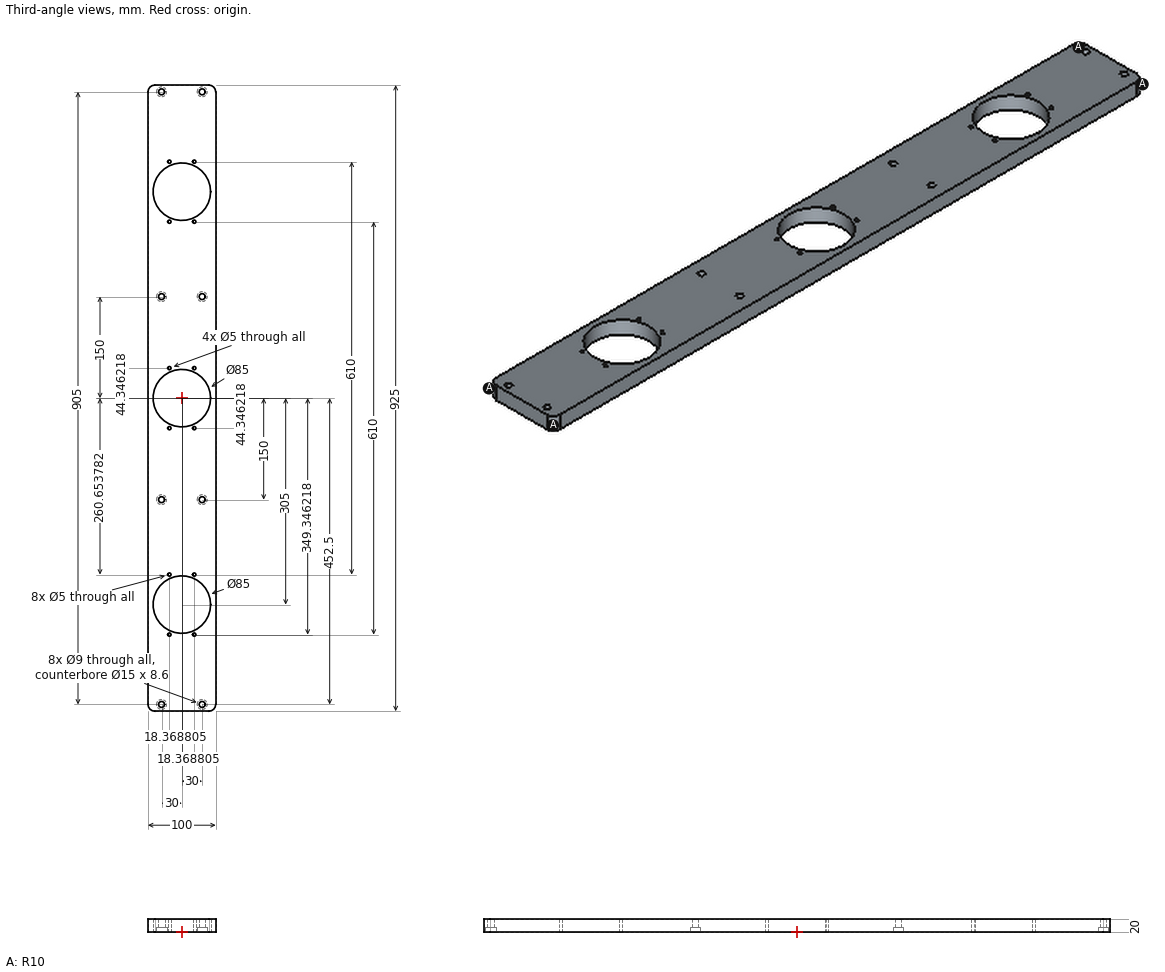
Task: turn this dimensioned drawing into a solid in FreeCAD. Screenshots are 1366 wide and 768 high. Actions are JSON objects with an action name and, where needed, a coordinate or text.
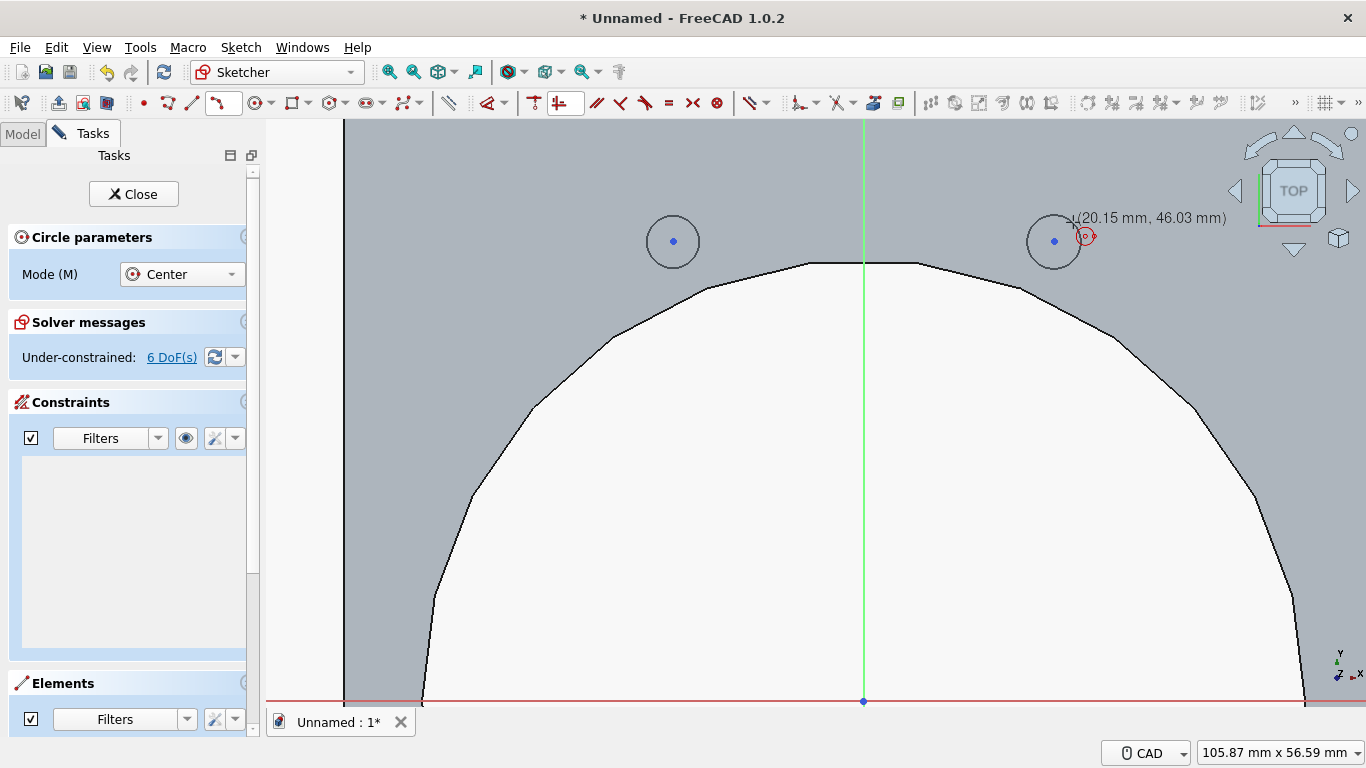
{"action": "scroll", "coordinate": [680, 245], "scroll_direction": "down", "scroll_amount": 5}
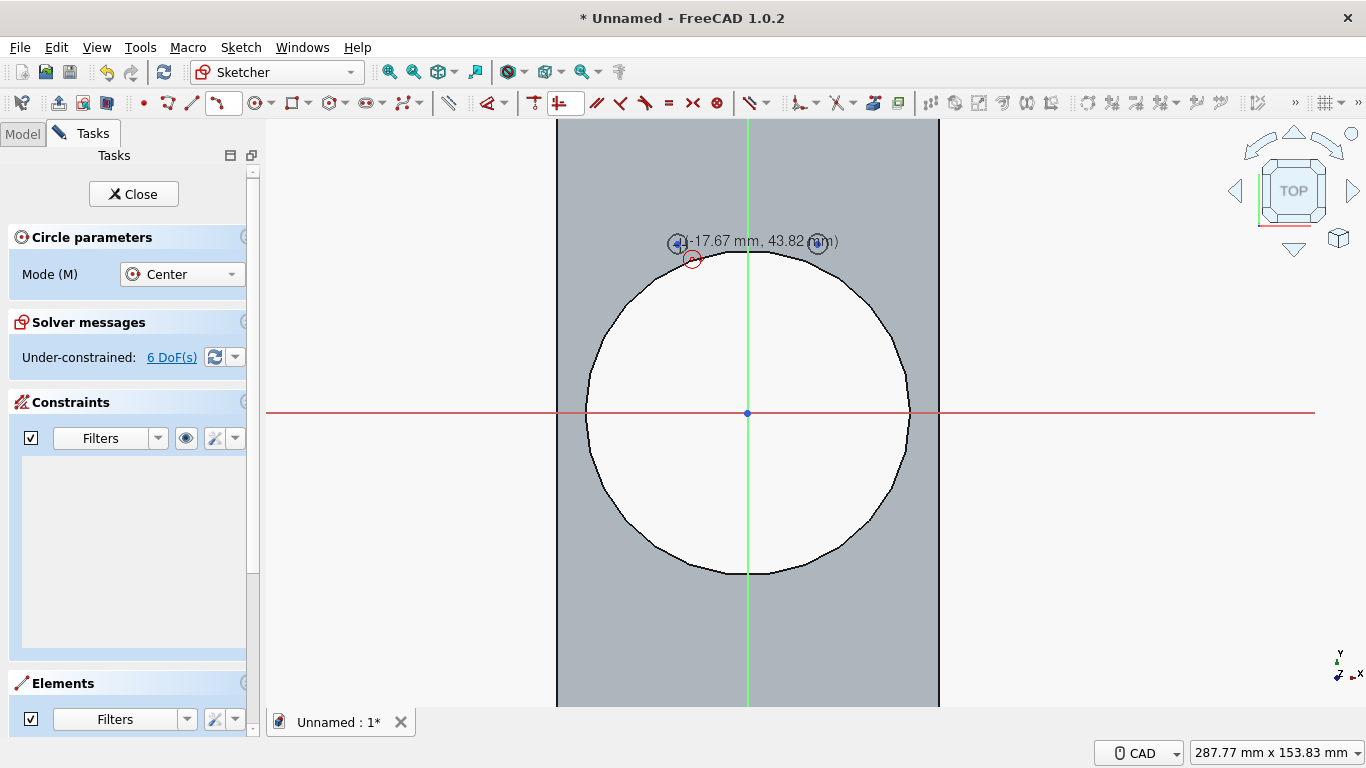
{"action": "scroll", "coordinate": [818, 583], "scroll_direction": "up", "scroll_amount": 5}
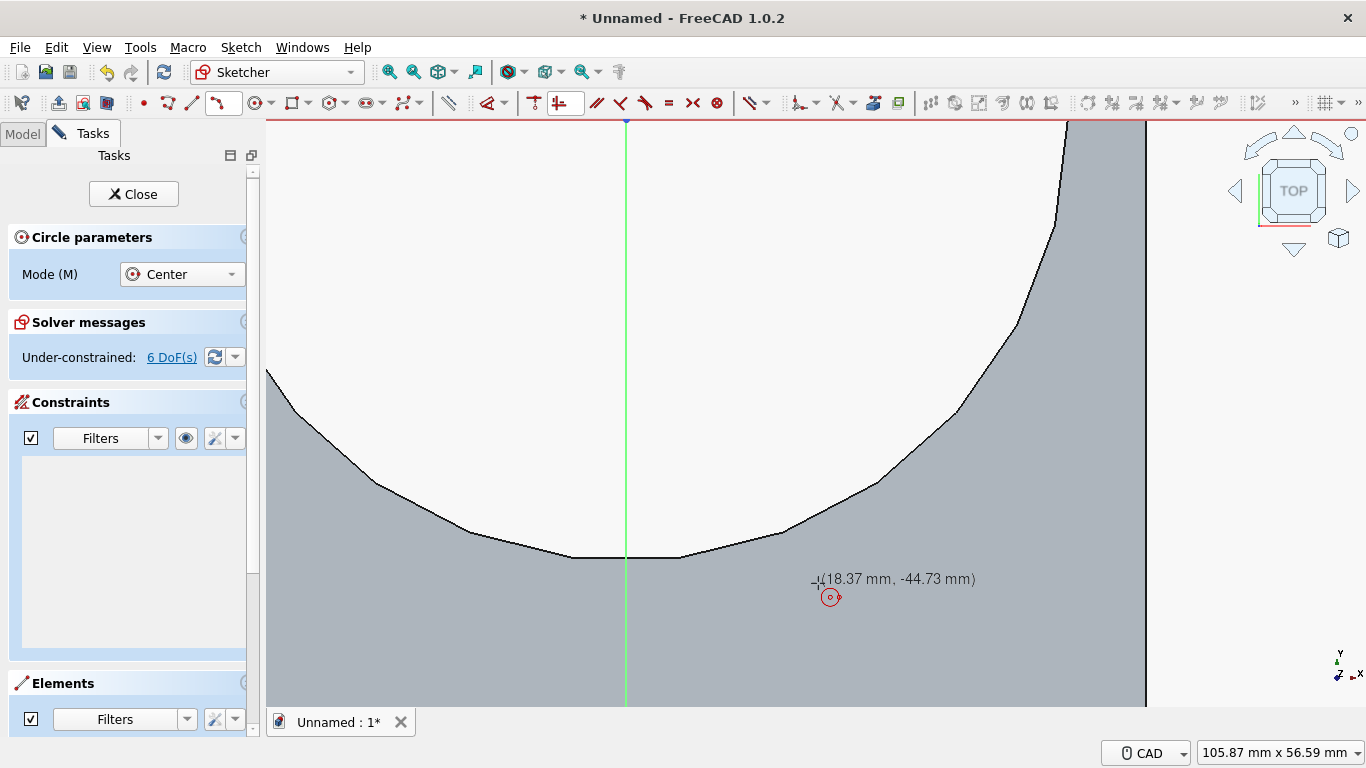
{"action": "left_click", "coordinate": [817, 580]}
{"action": "left_click", "coordinate": [835, 562]}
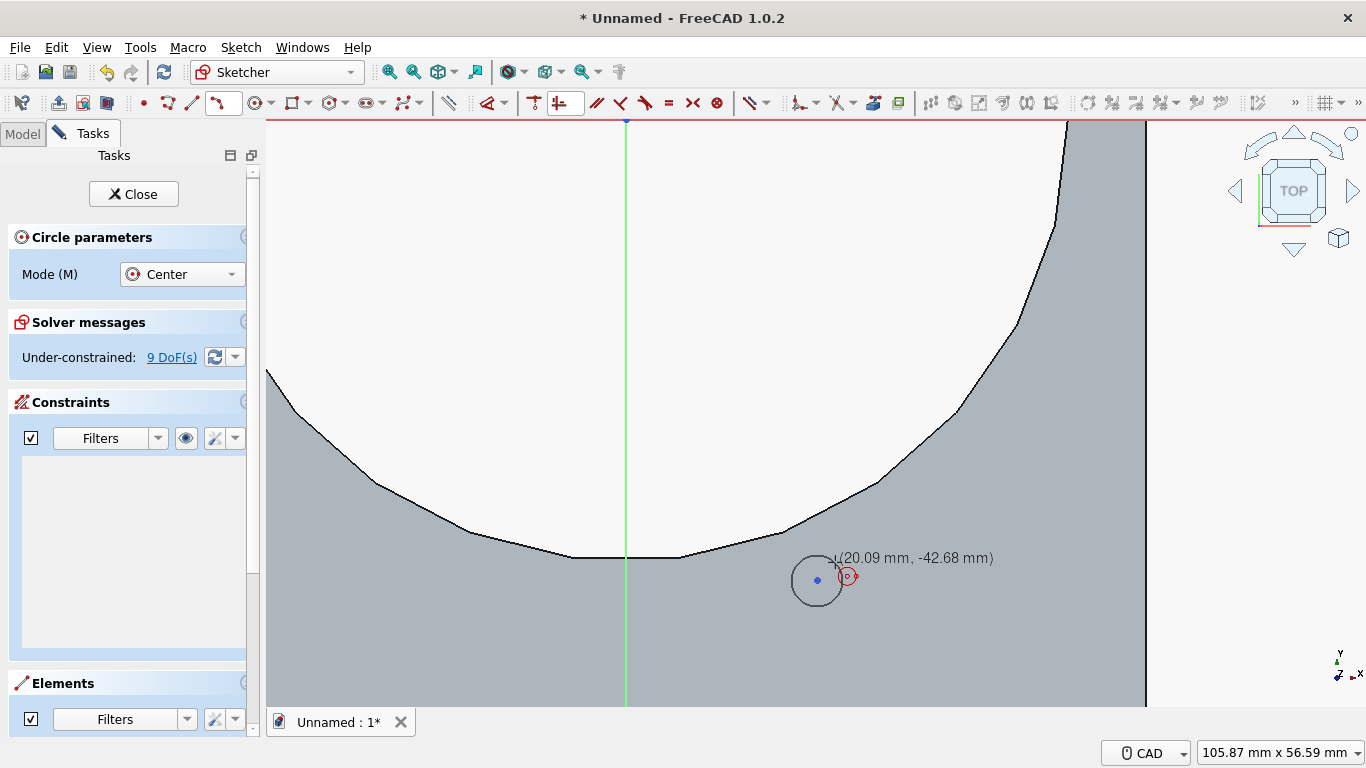
{"action": "left_click", "coordinate": [435, 580]}
{"action": "left_click", "coordinate": [454, 562]}
{"action": "key", "text": "Escape"}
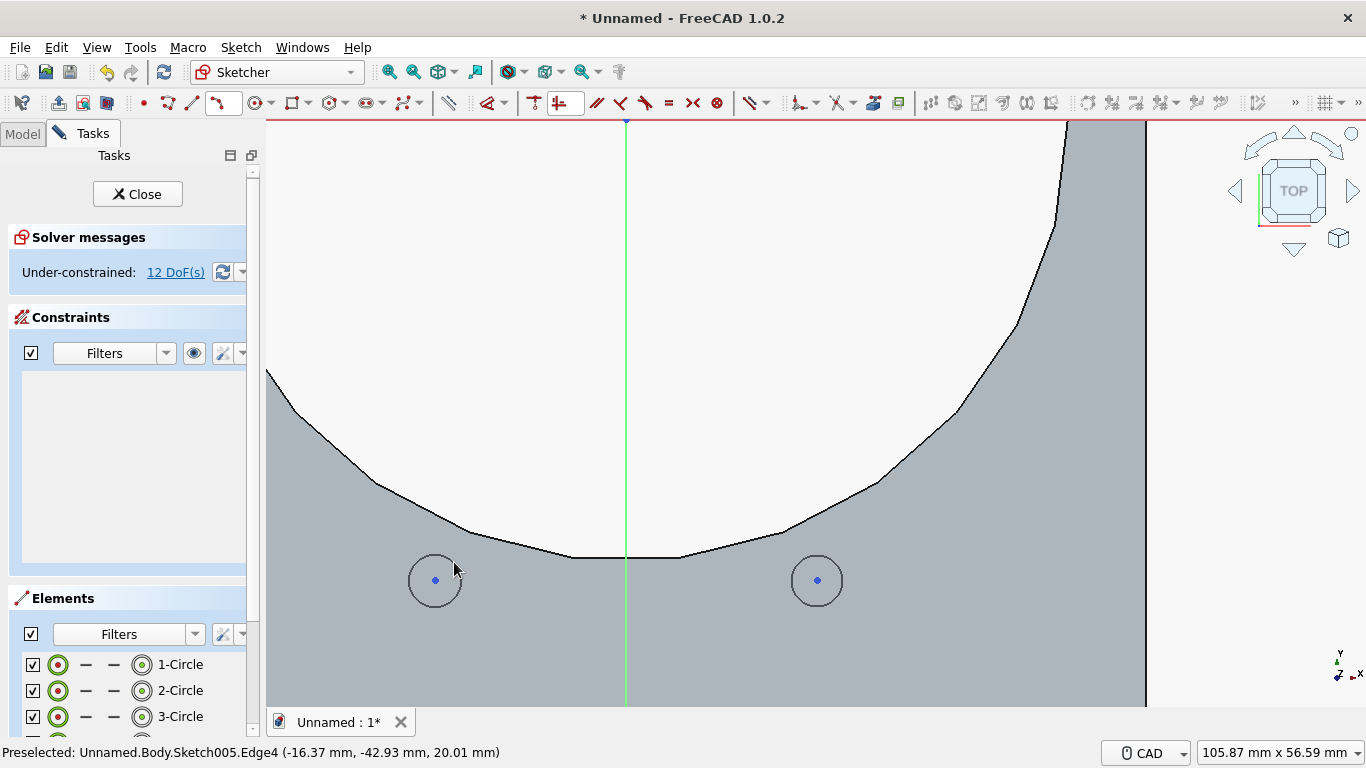
{"action": "scroll", "coordinate": [818, 584], "scroll_direction": "down", "scroll_amount": 5}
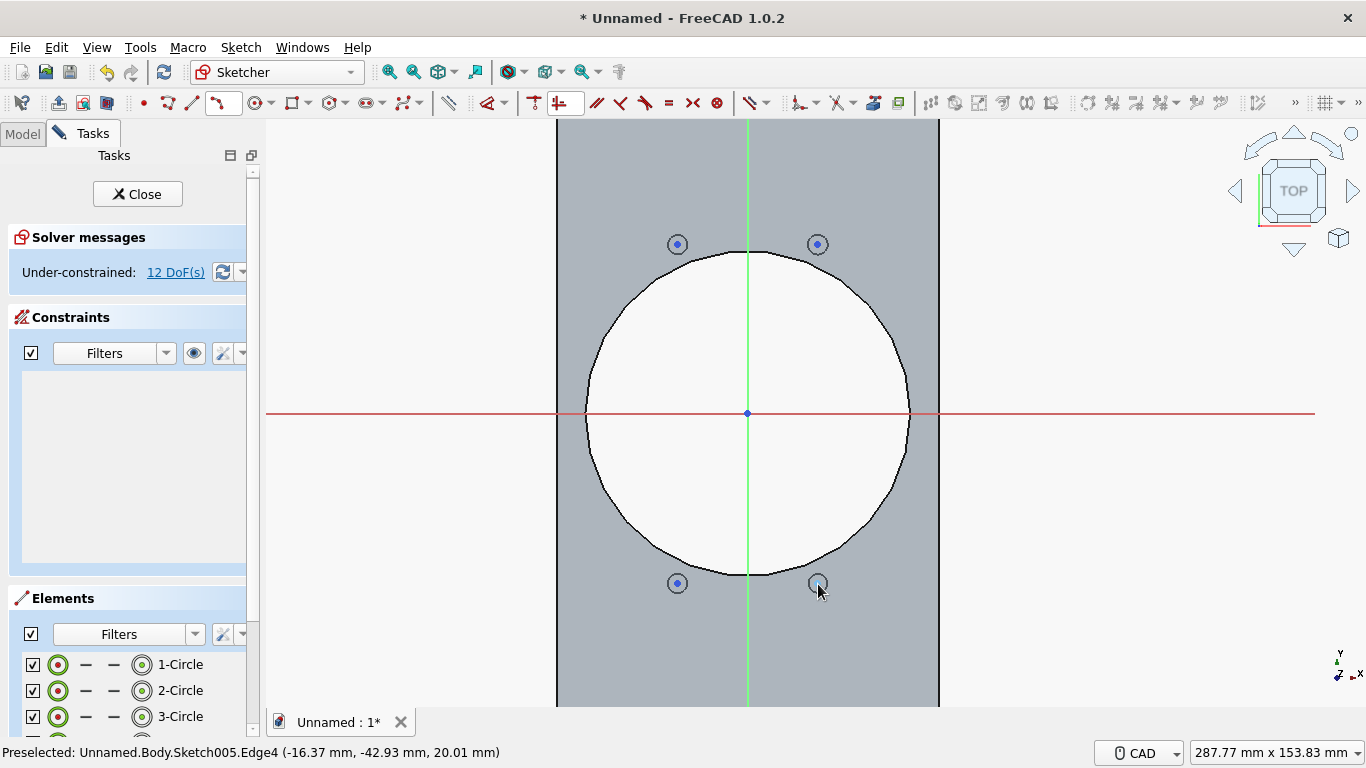
{"action": "scroll", "coordinate": [684, 238], "scroll_direction": "up", "scroll_amount": 2}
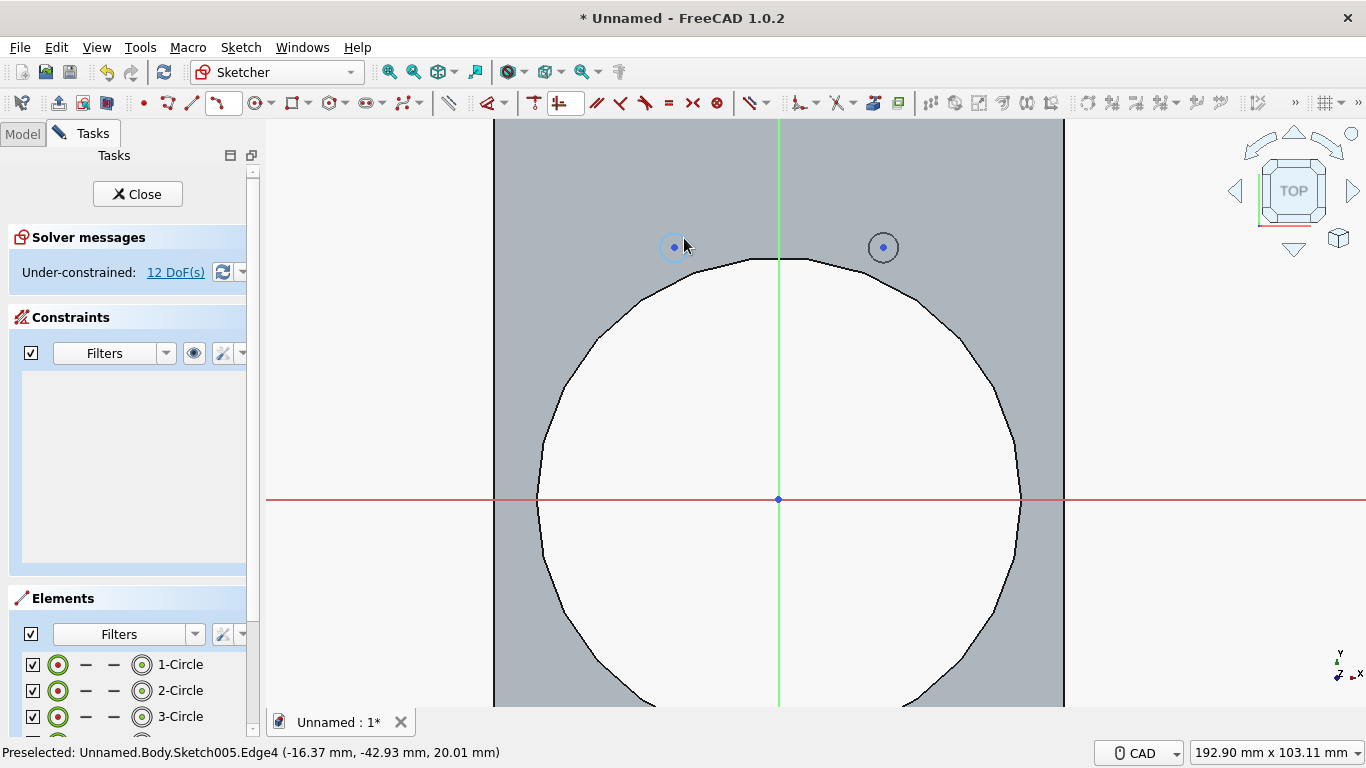
{"action": "left_click", "coordinate": [684, 238]}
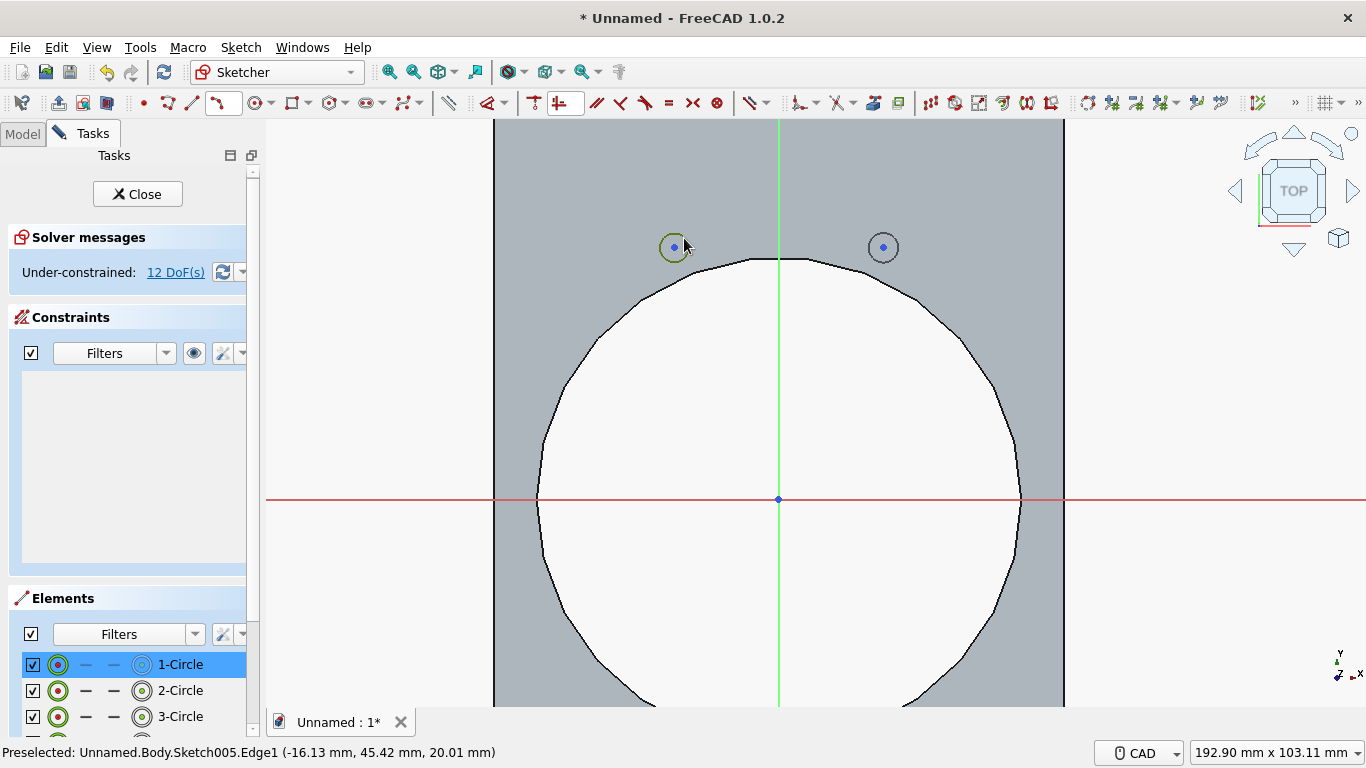
{"action": "left_click", "coordinate": [894, 237]}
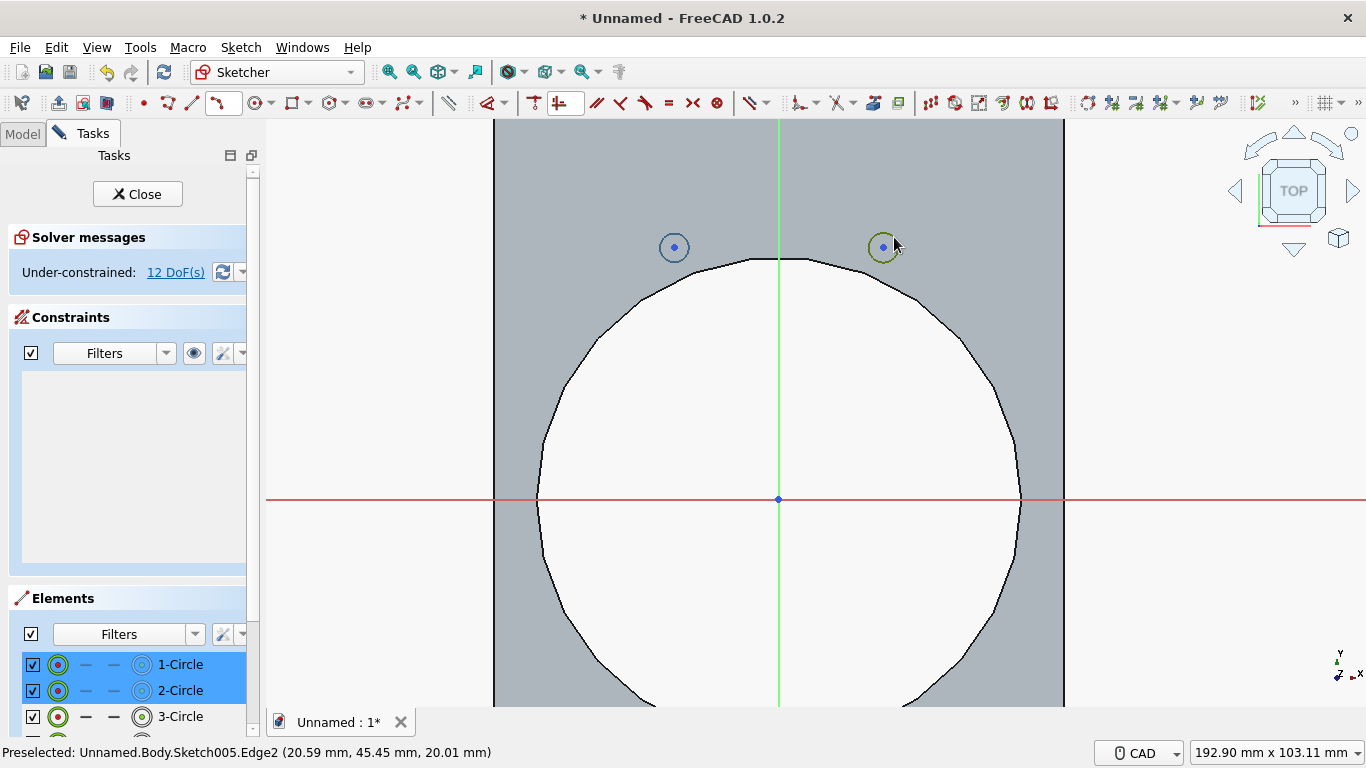
{"action": "scroll", "coordinate": [684, 236], "scroll_direction": "down", "scroll_amount": 2}